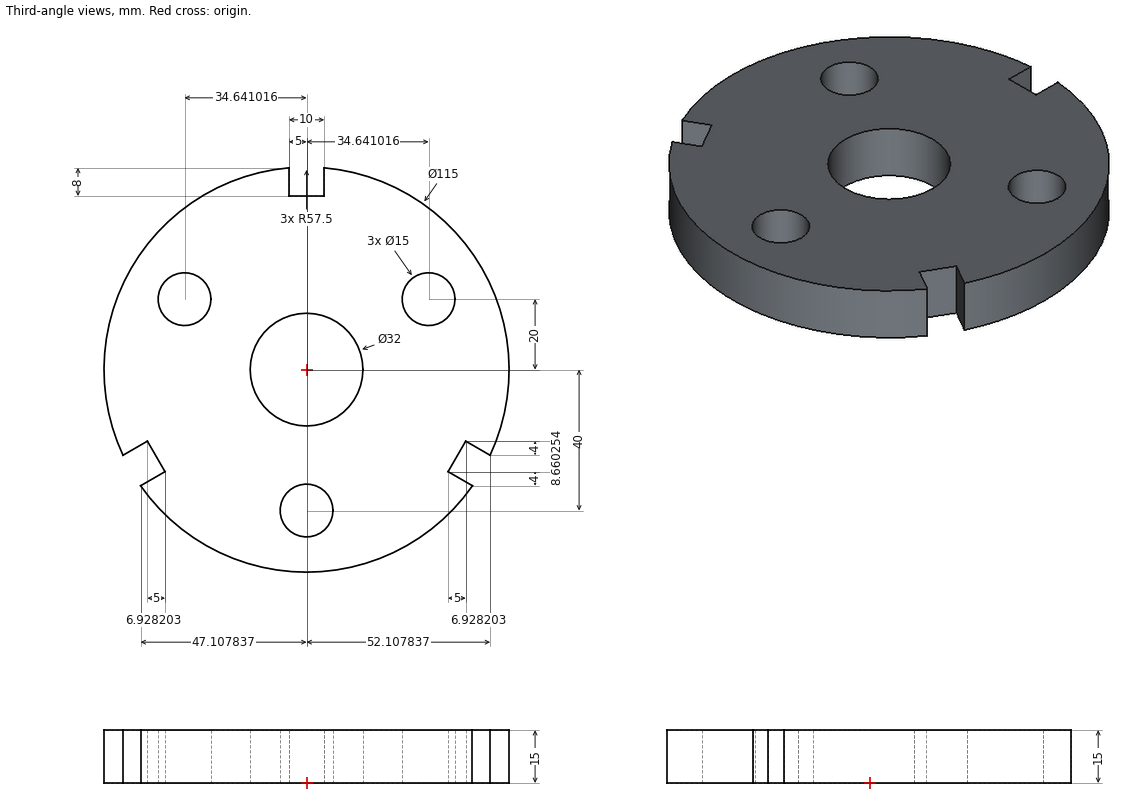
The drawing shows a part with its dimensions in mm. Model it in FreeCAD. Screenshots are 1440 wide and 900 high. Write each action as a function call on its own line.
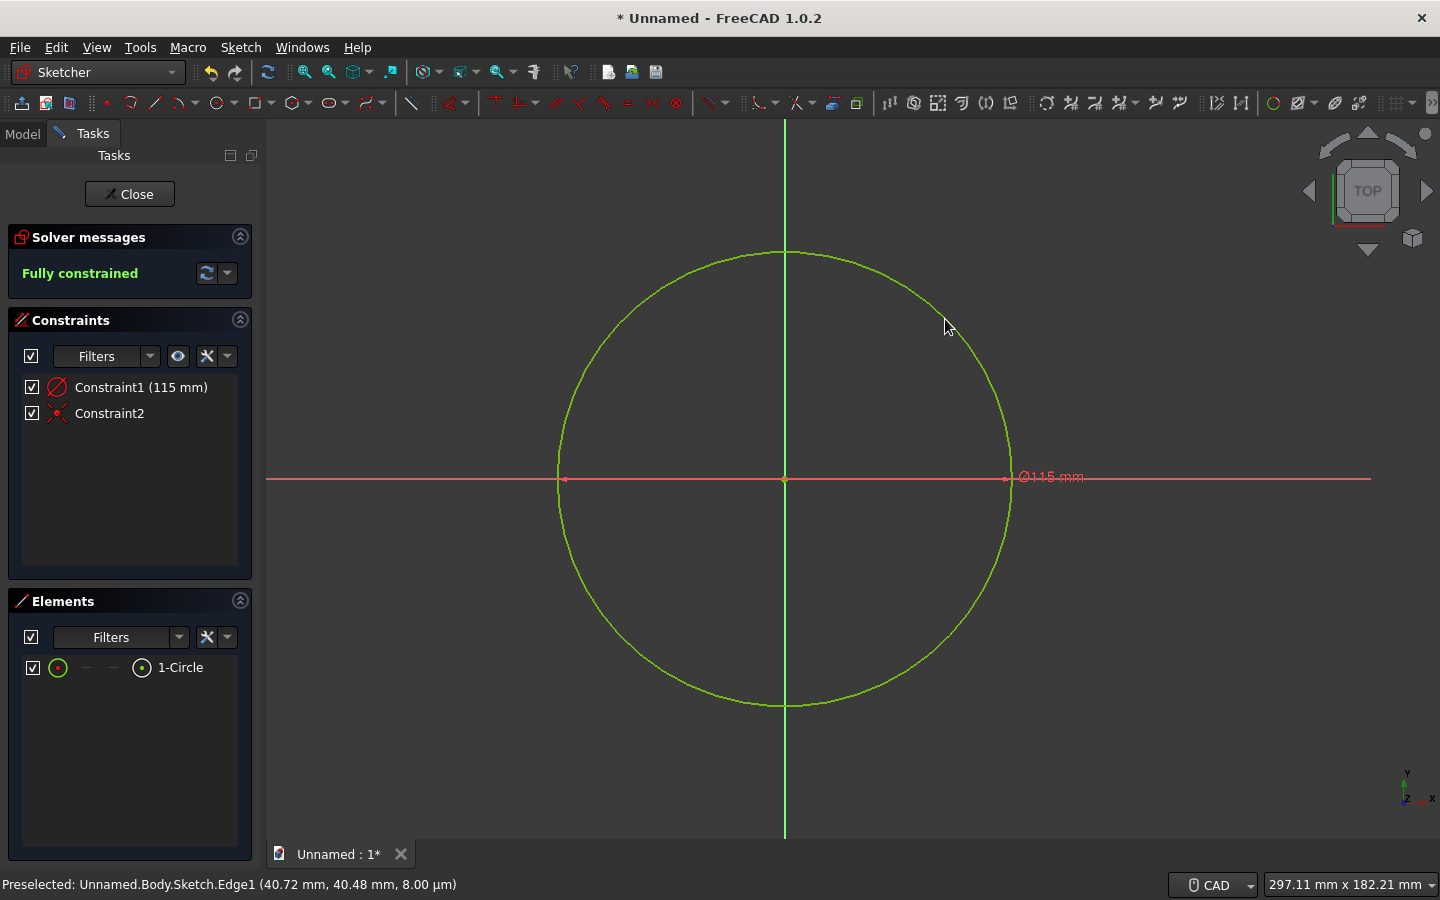
click(130, 194)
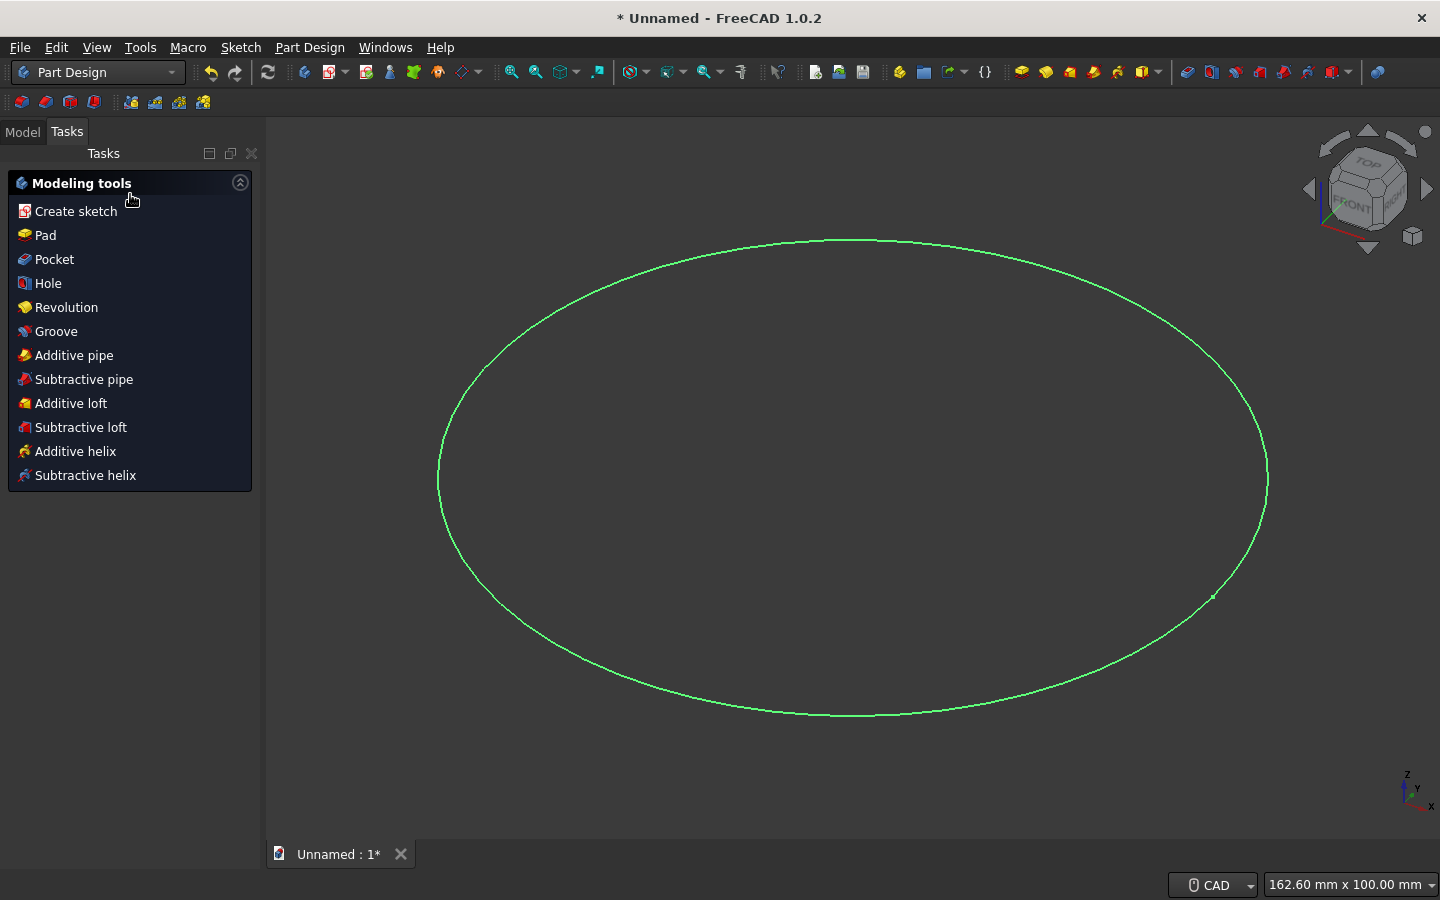
click(1022, 72)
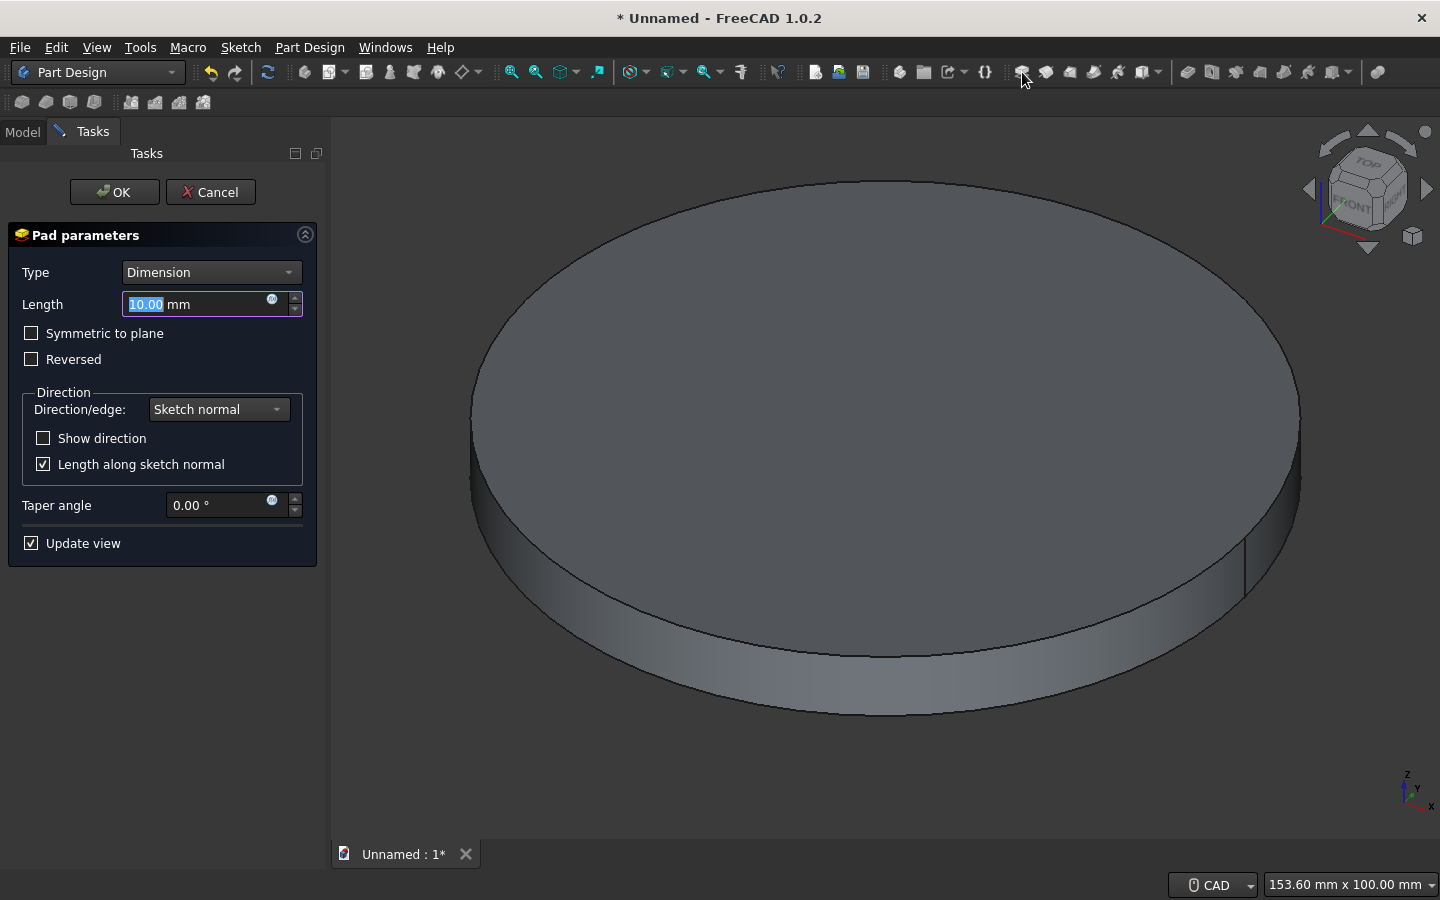
text(15)
key(Tab)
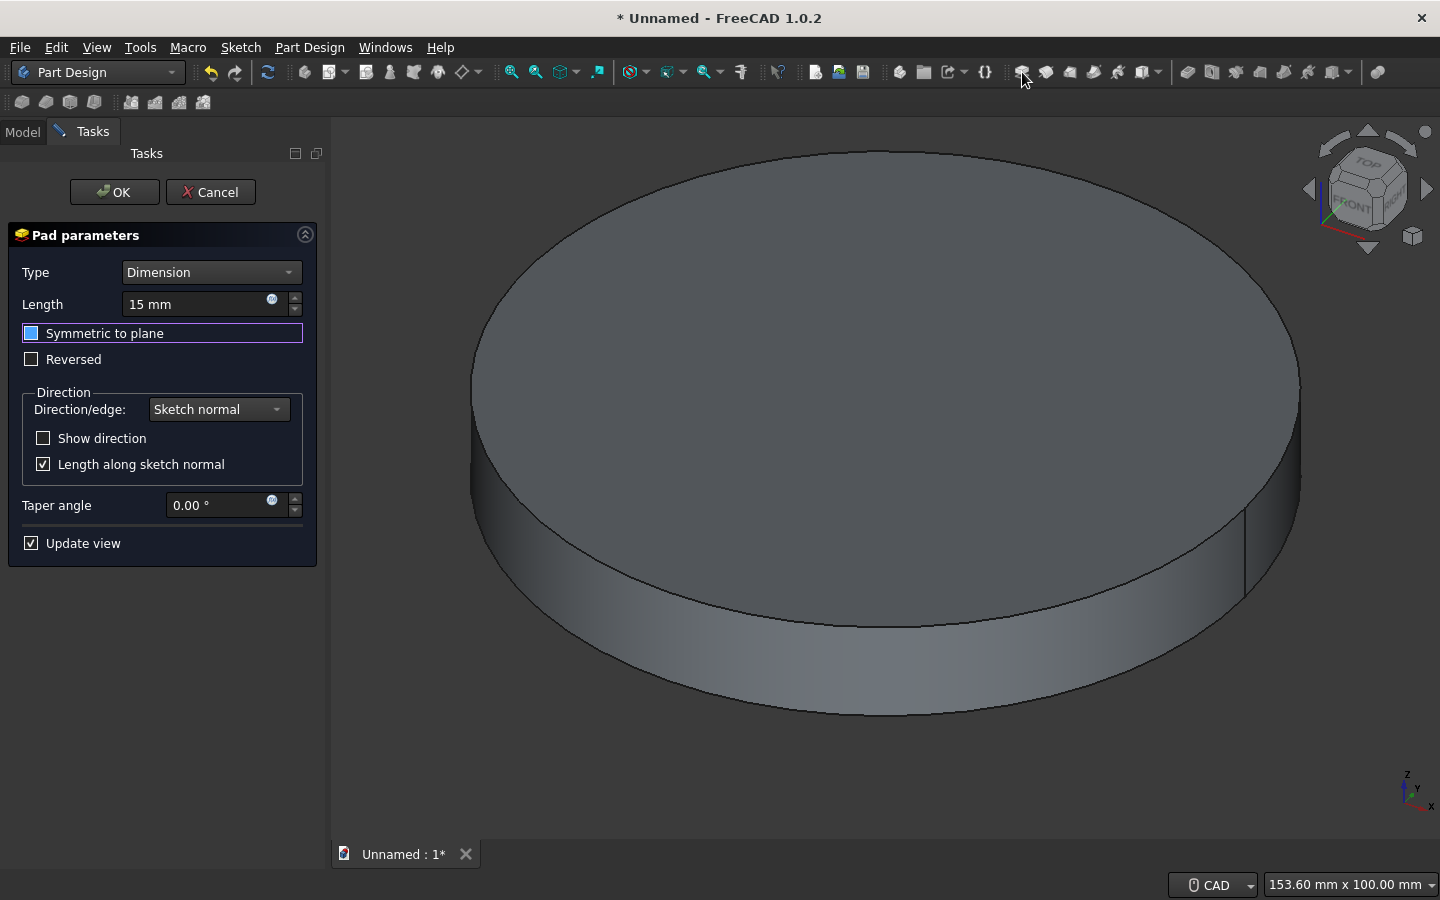
click(115, 192)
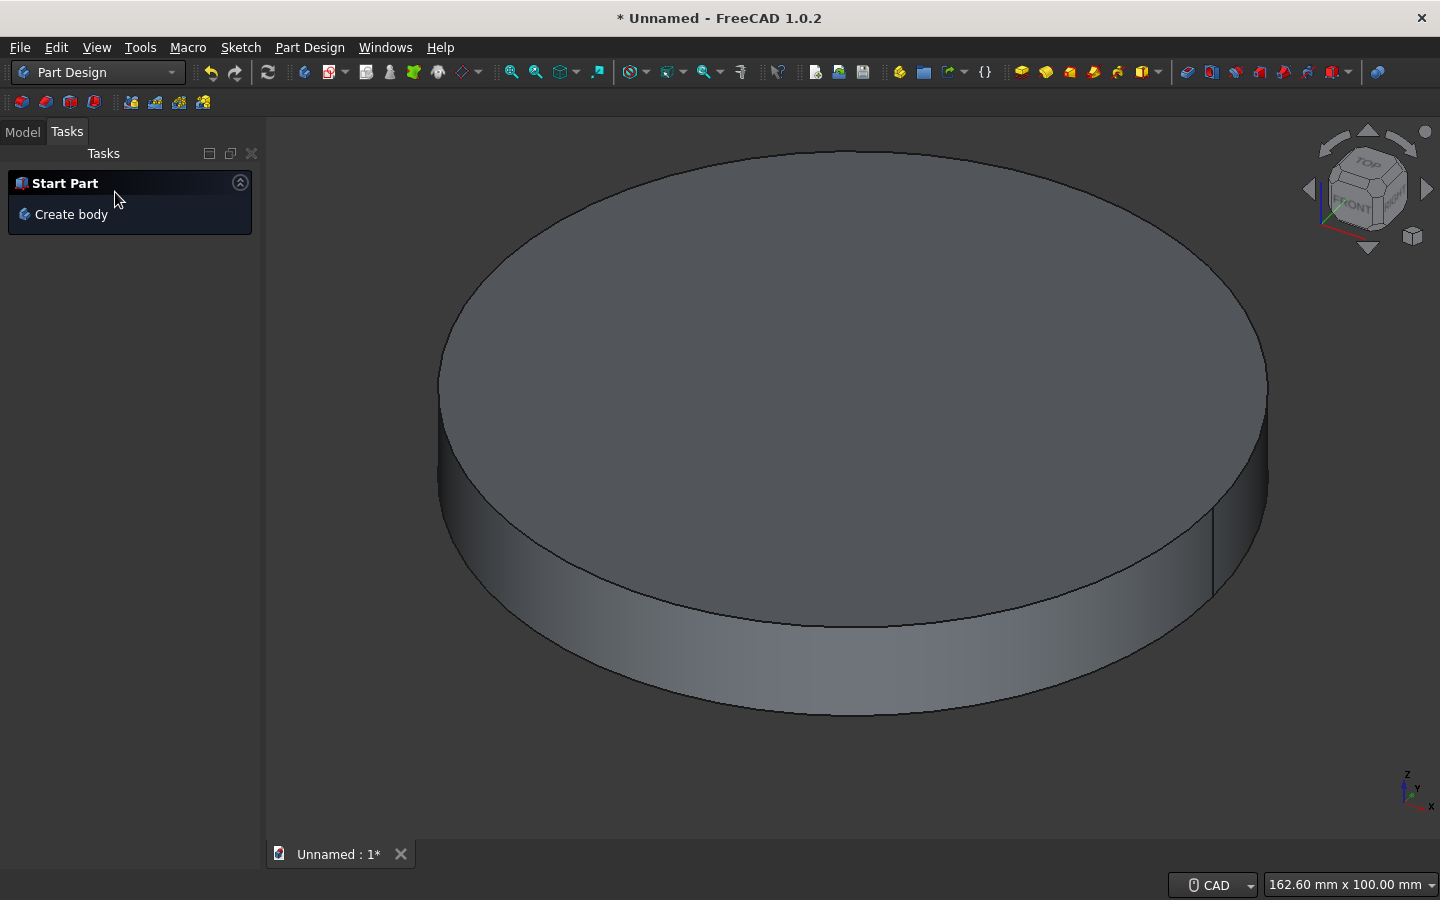
key(v)
key(f)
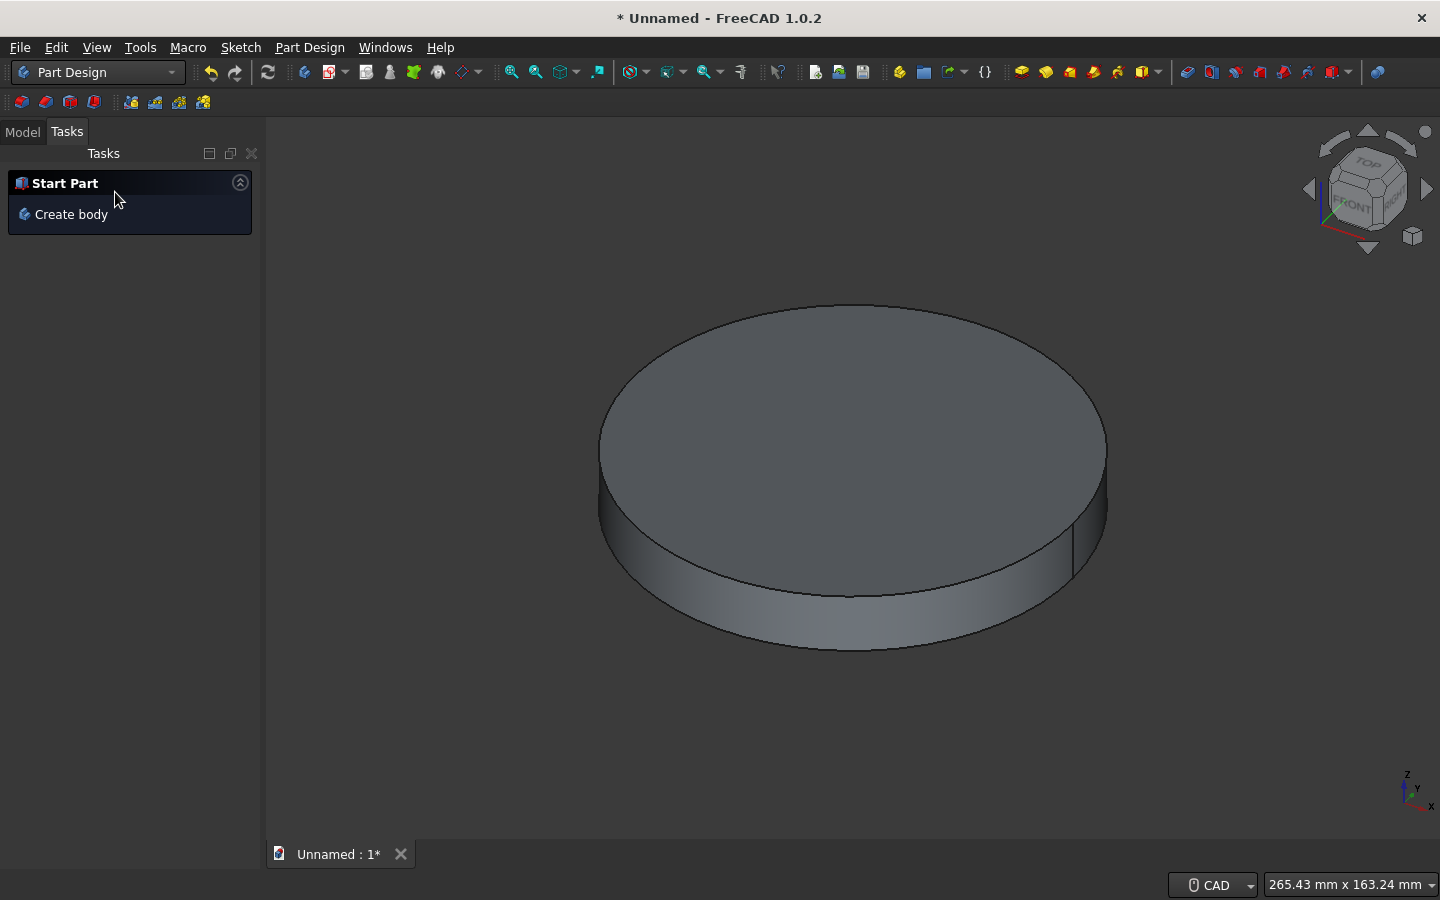
click(853, 450)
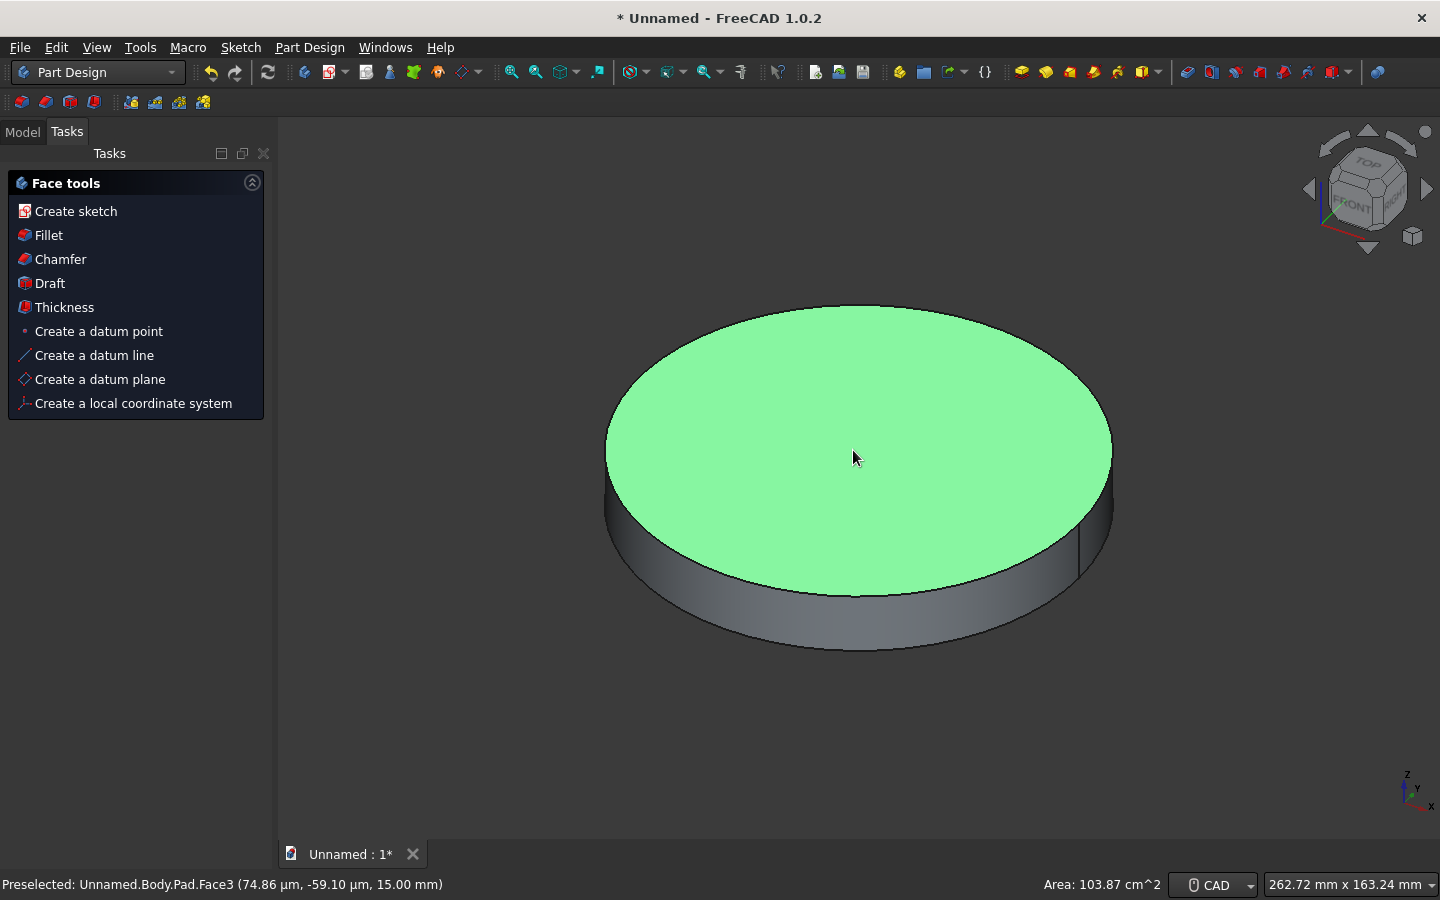
click(330, 72)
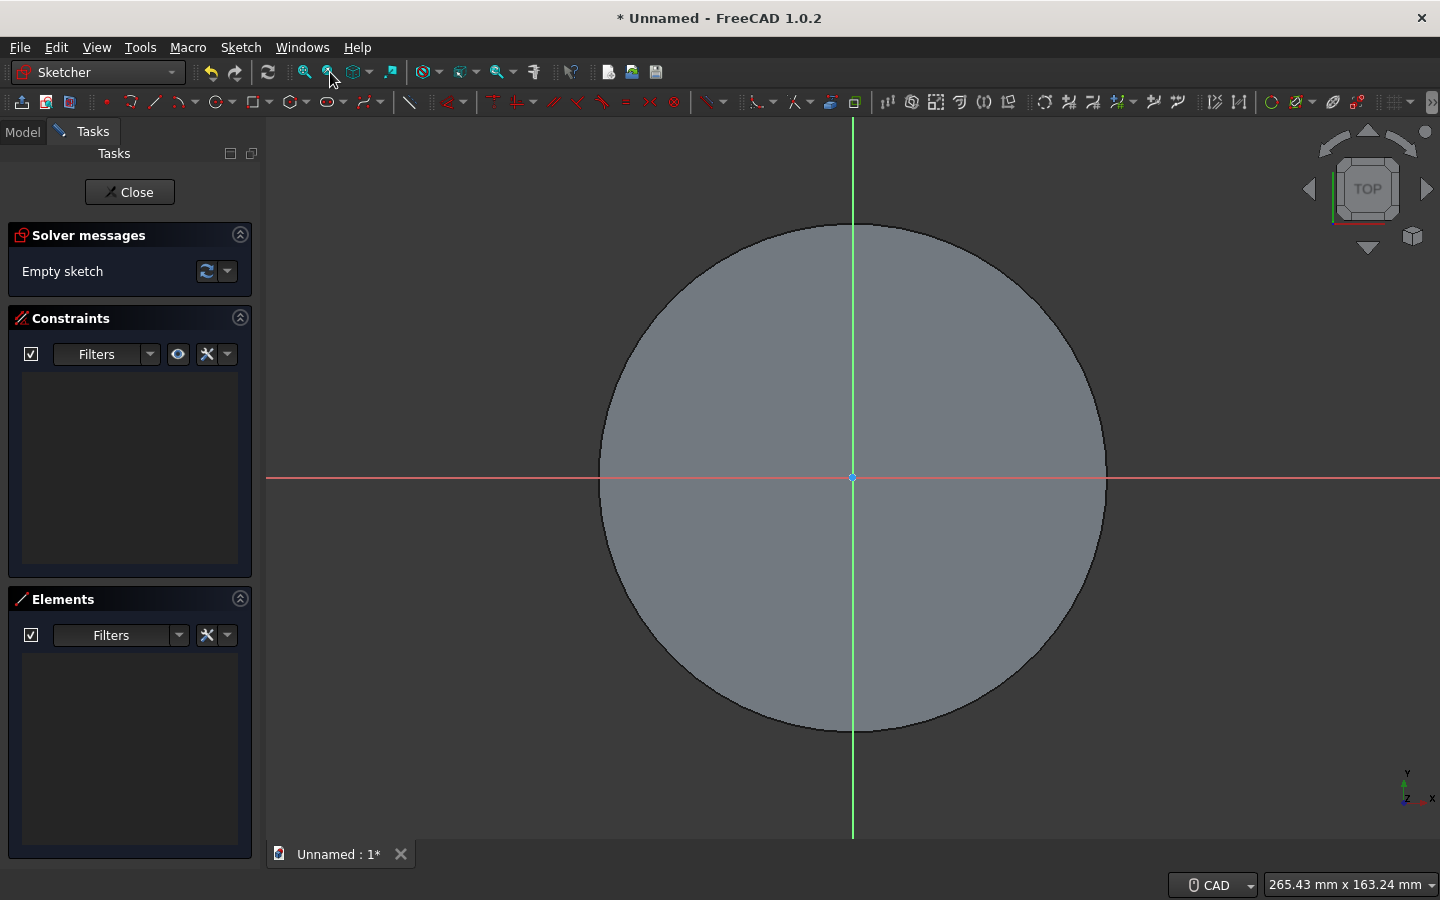
scroll(992, 612, up, 2)